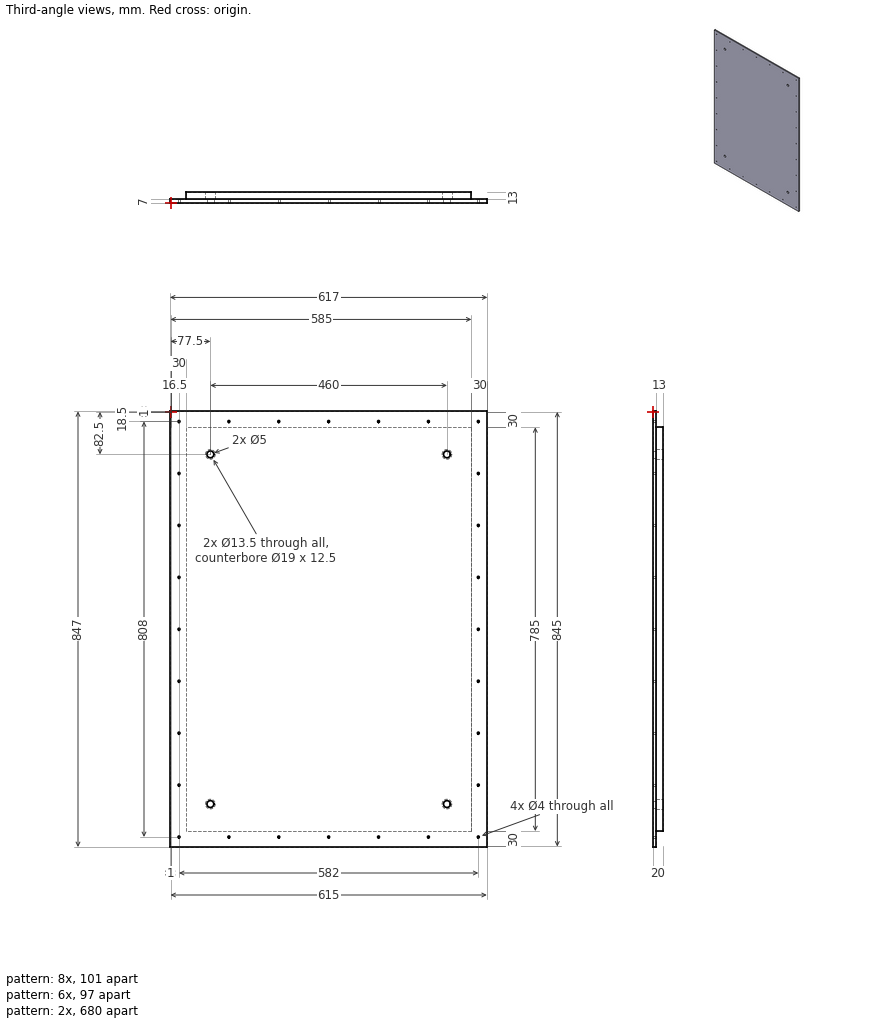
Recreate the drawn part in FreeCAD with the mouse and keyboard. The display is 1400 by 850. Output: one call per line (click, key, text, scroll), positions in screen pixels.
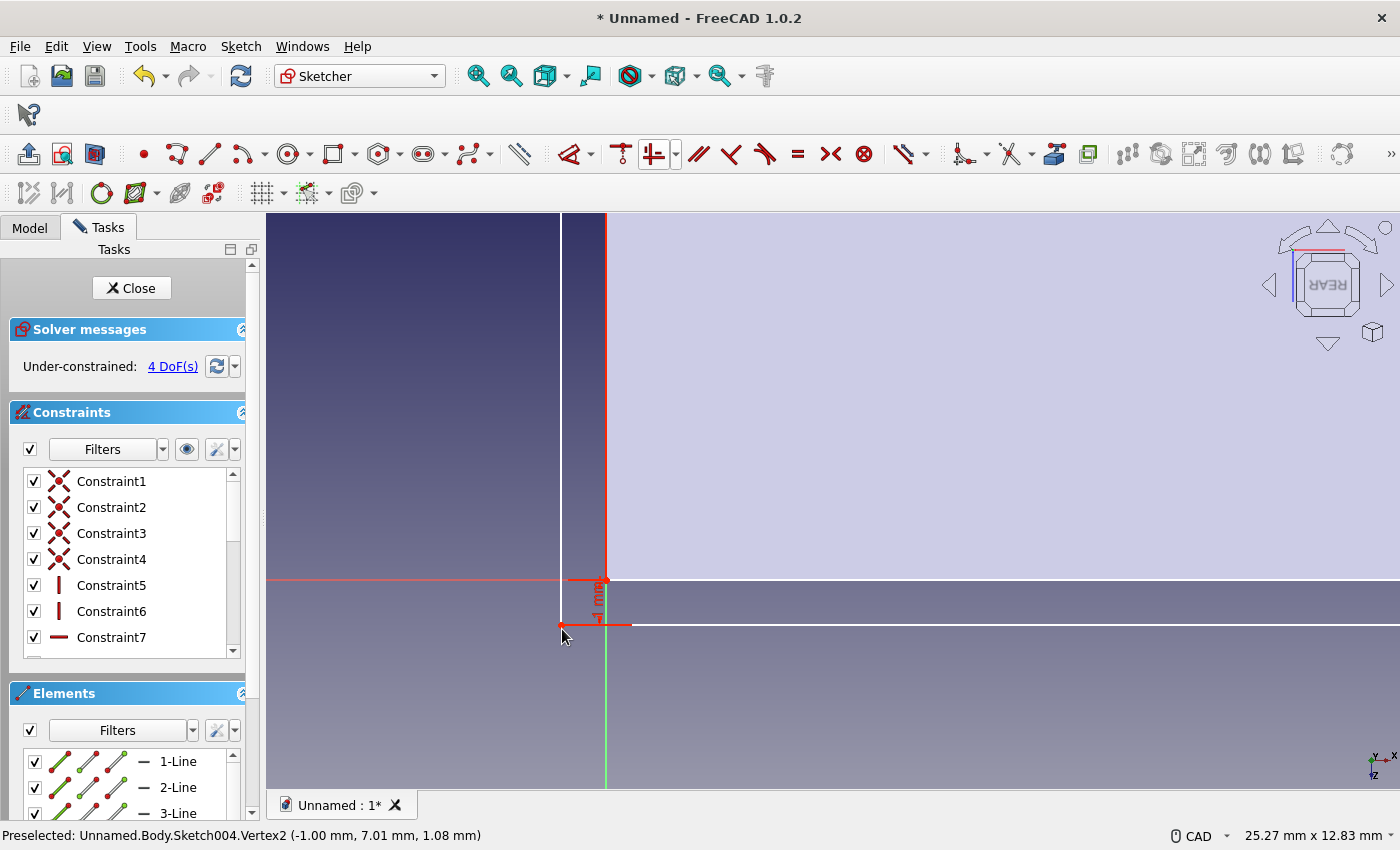
scroll(764, 501, down, 15)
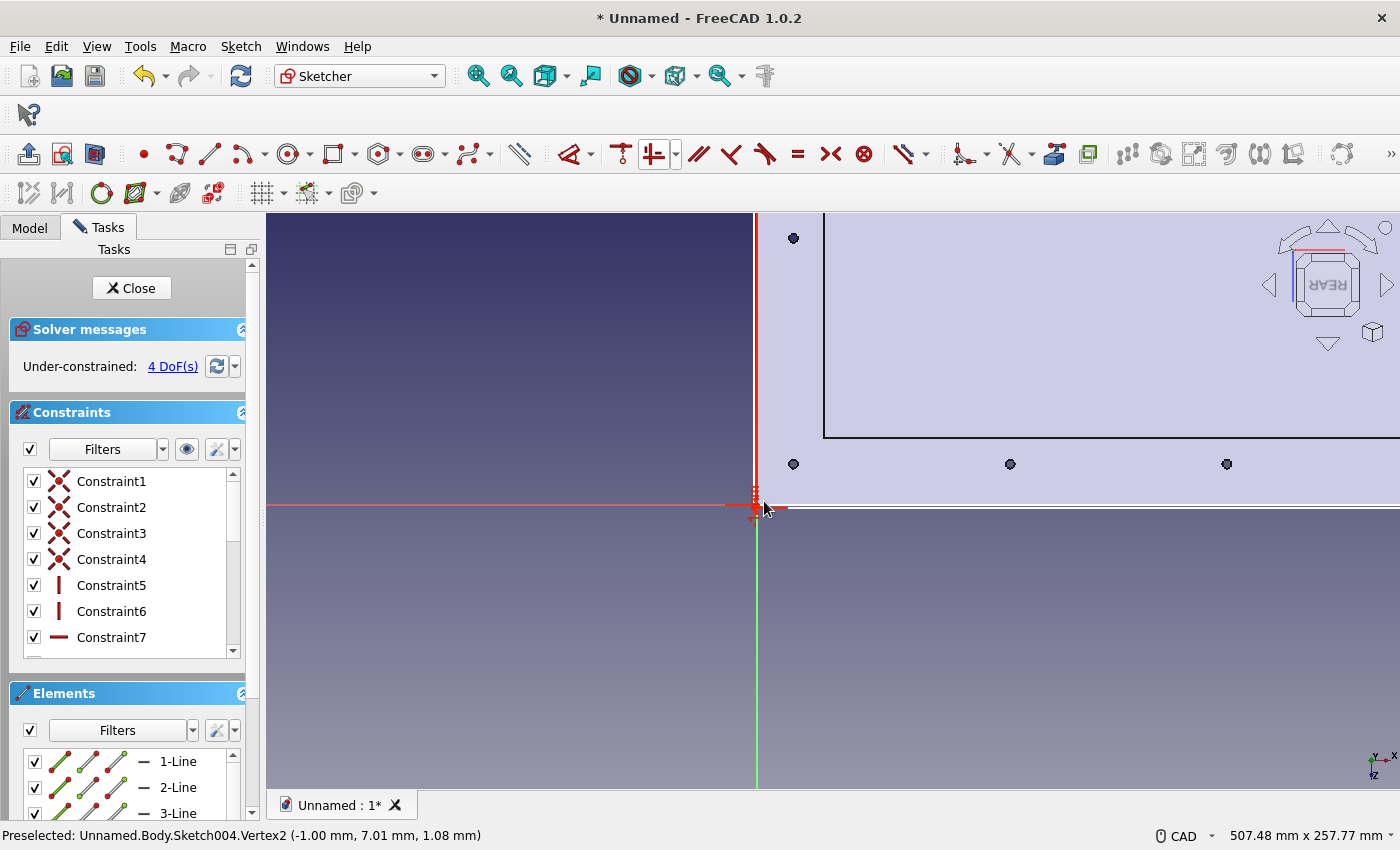
scroll(593, 739, down, 8)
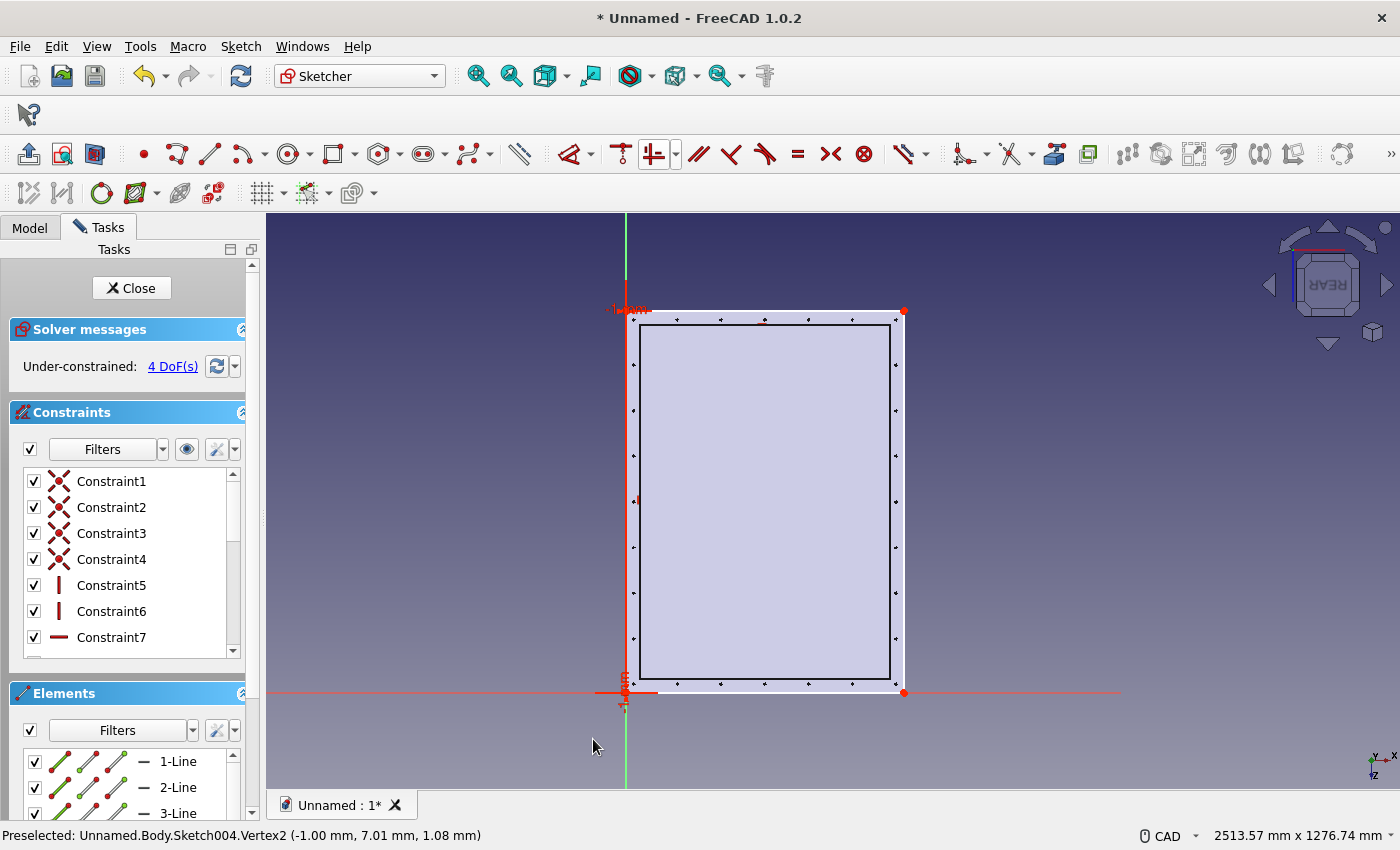
scroll(626, 426, up, 15)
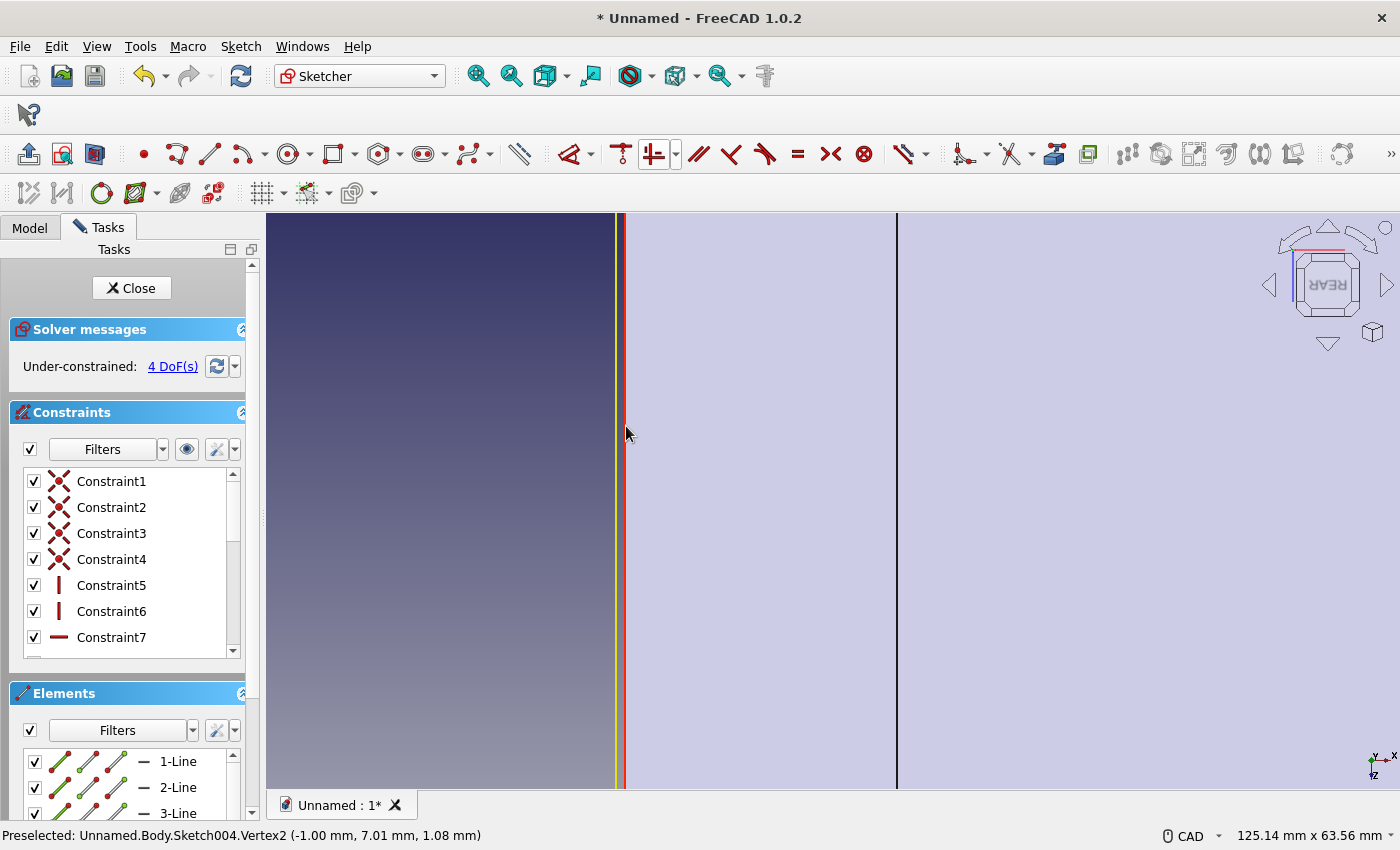
click(616, 410)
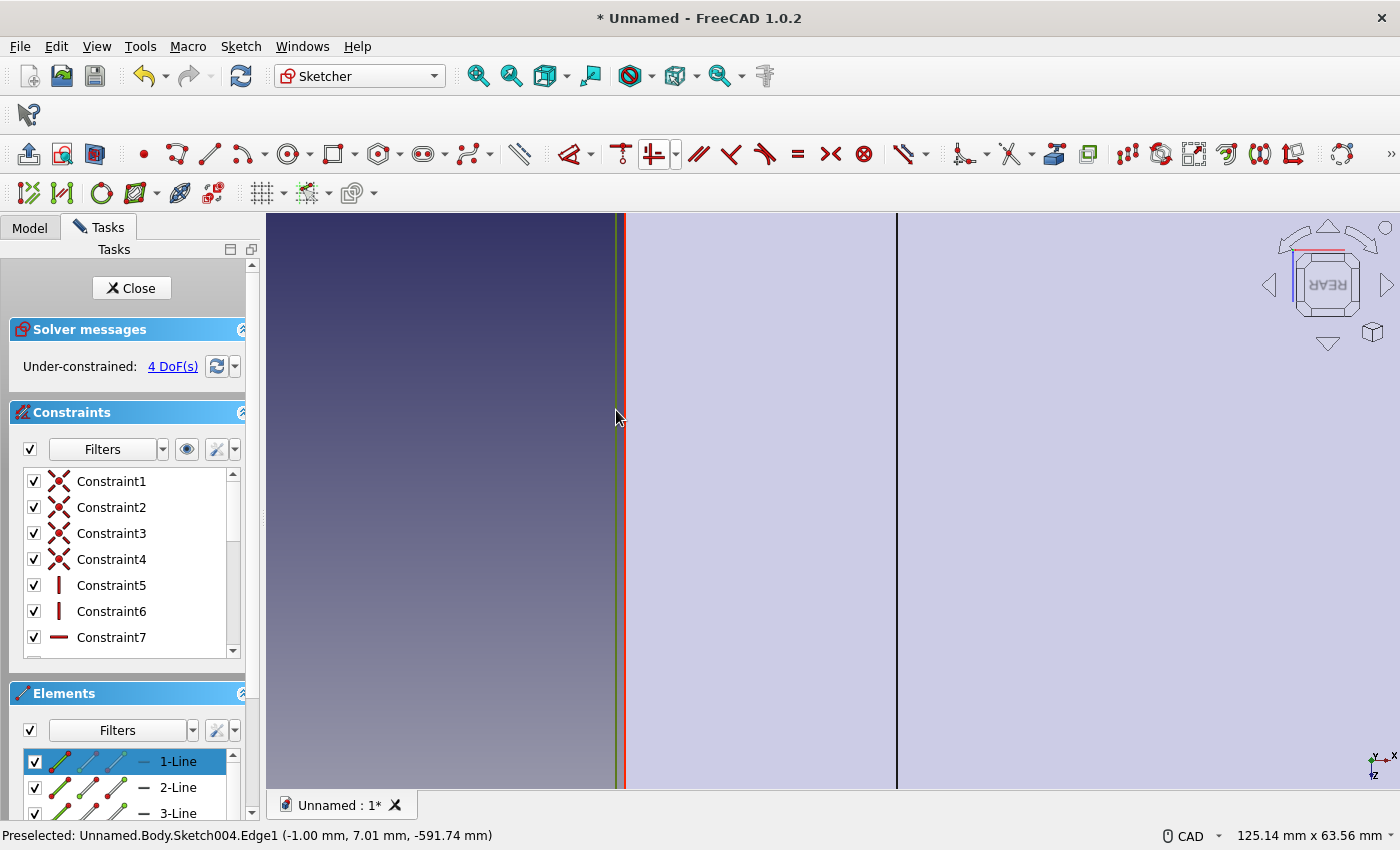
click(590, 154)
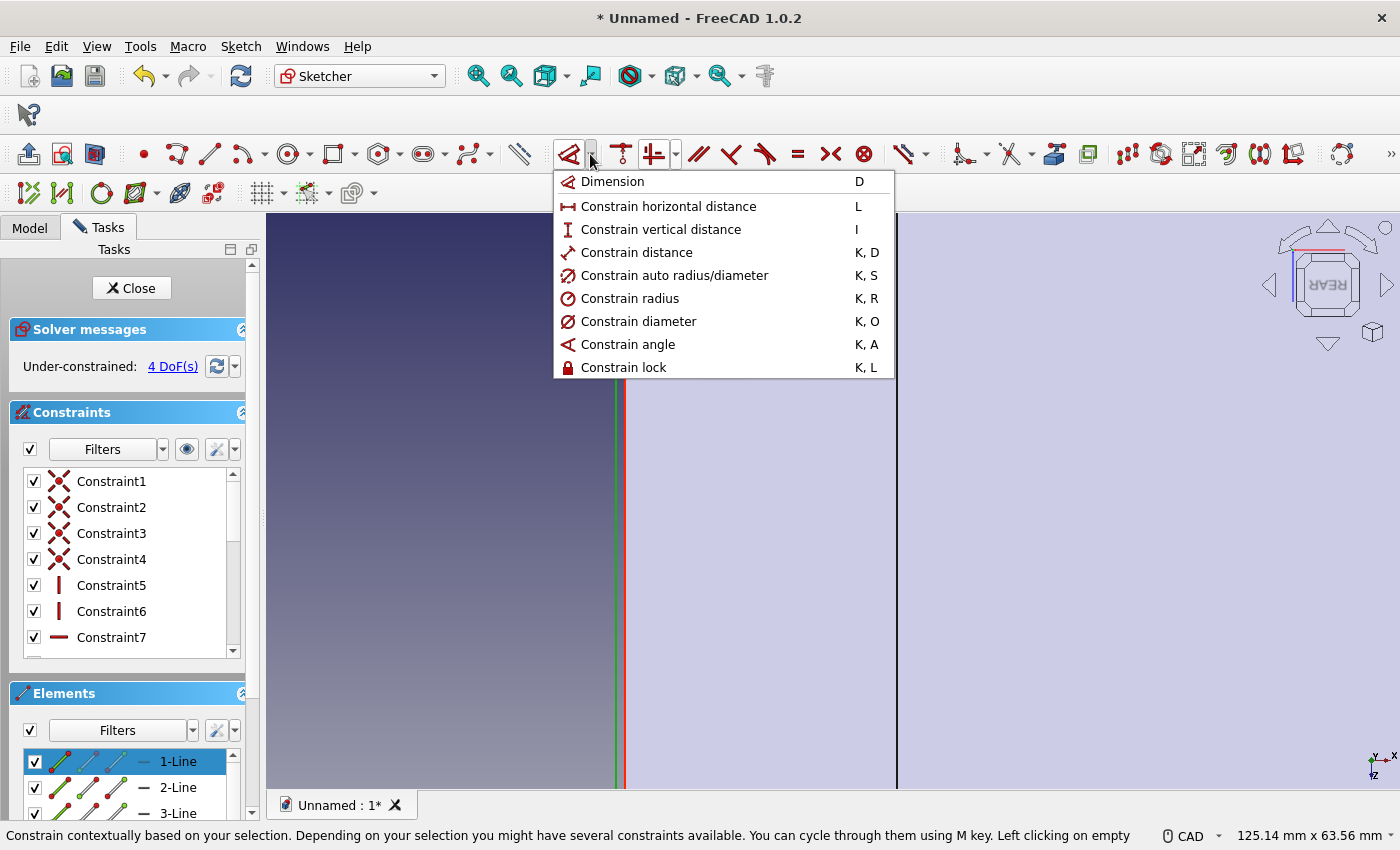
click(724, 230)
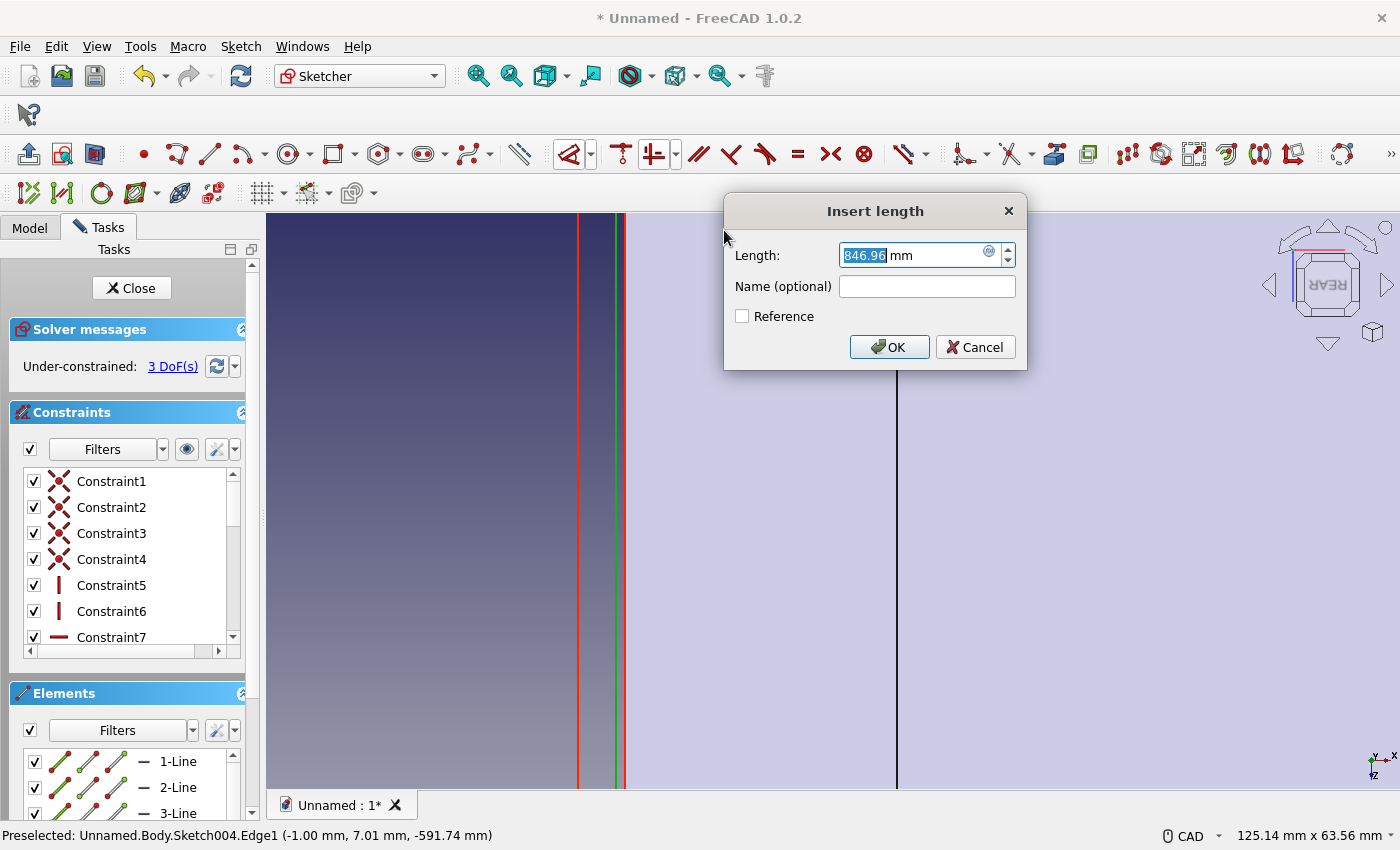
text(847)
key(Return)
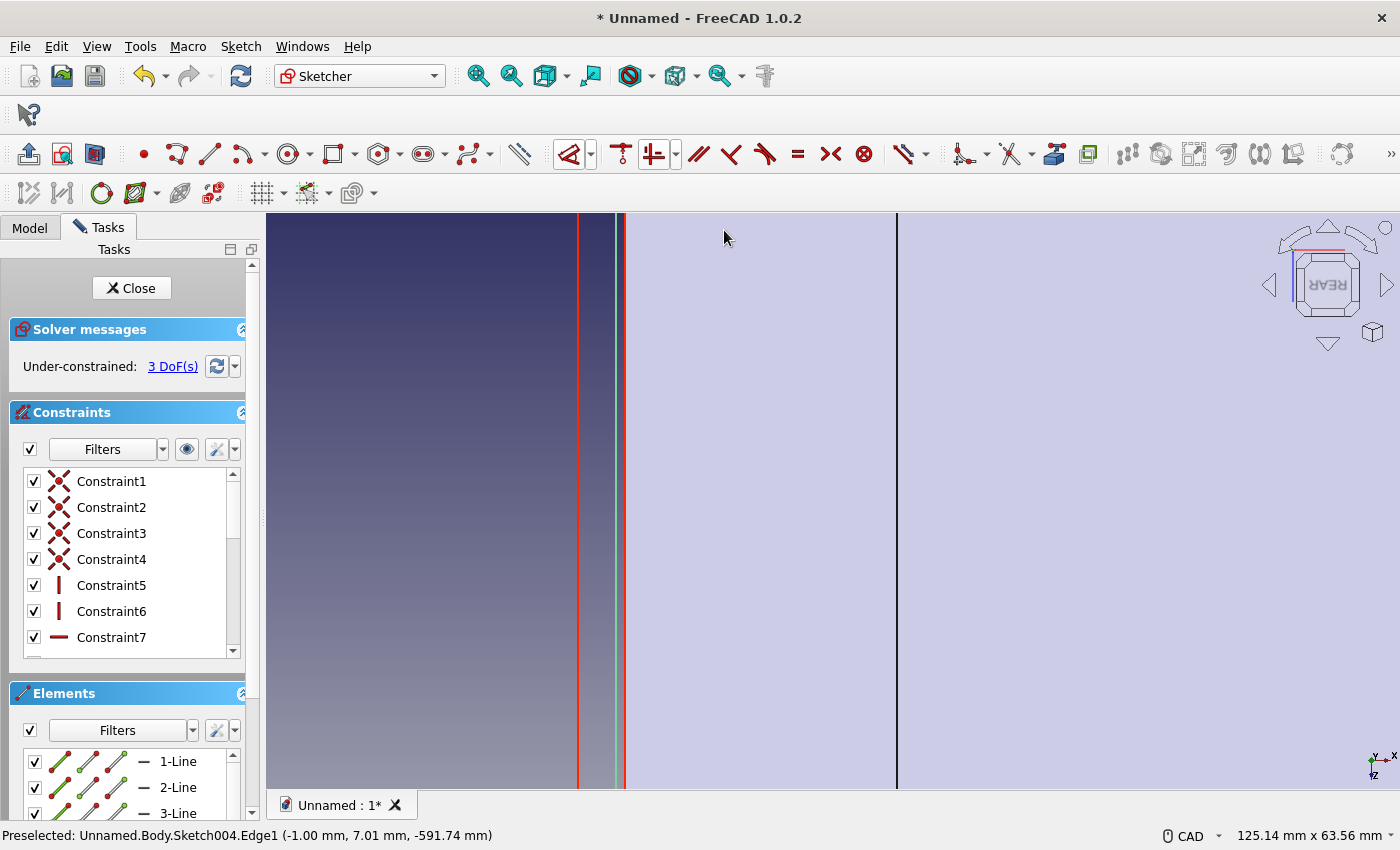
scroll(626, 425, down, 15)